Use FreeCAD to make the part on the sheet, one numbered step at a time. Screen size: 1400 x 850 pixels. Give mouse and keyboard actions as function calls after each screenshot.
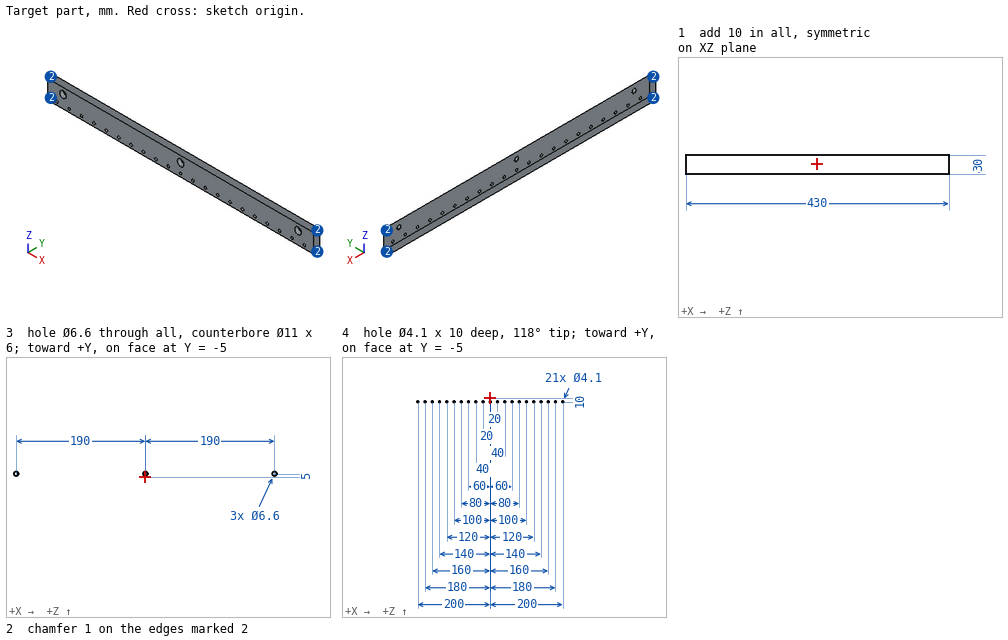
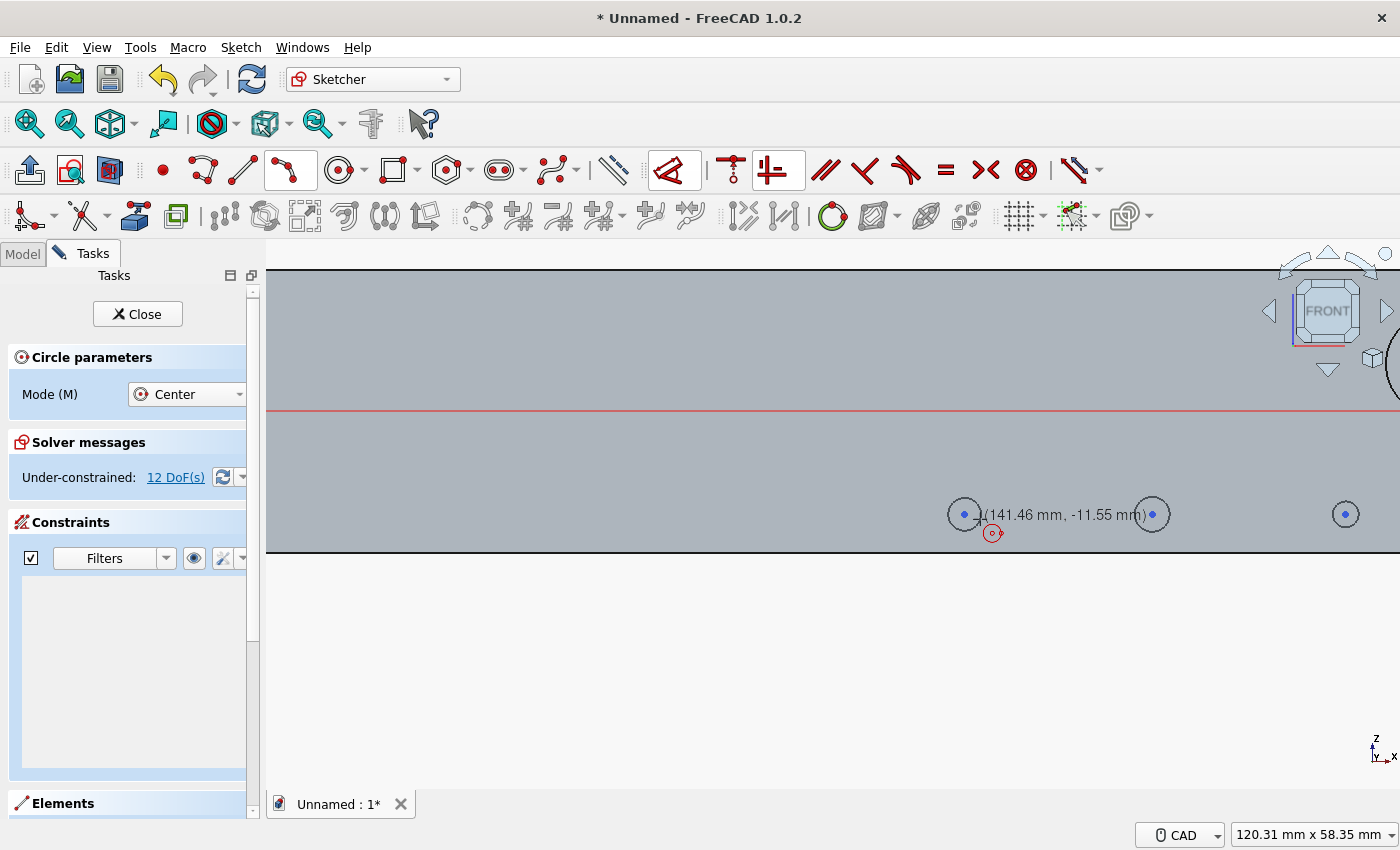
scroll(986, 523, down, 9)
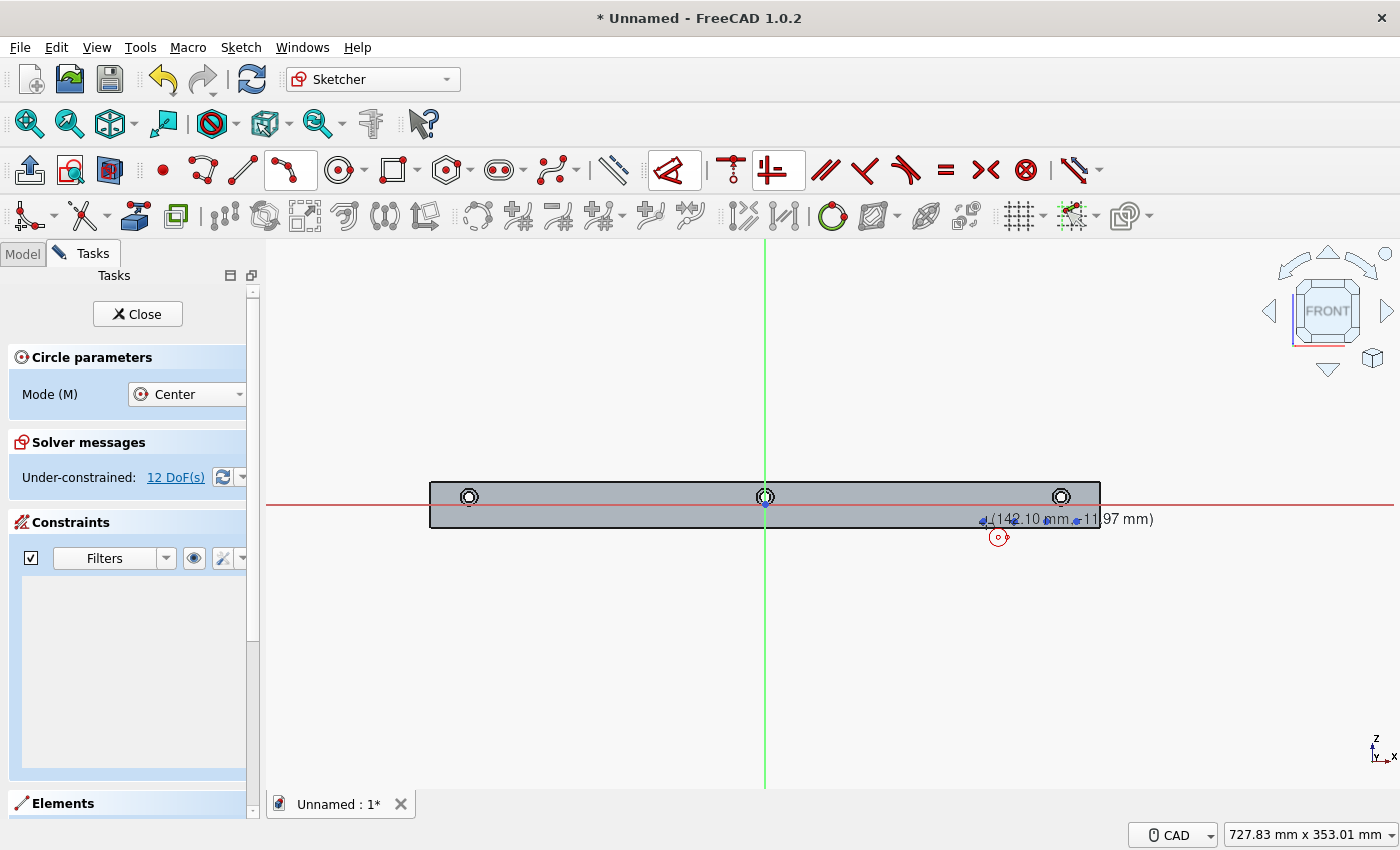
click(952, 521)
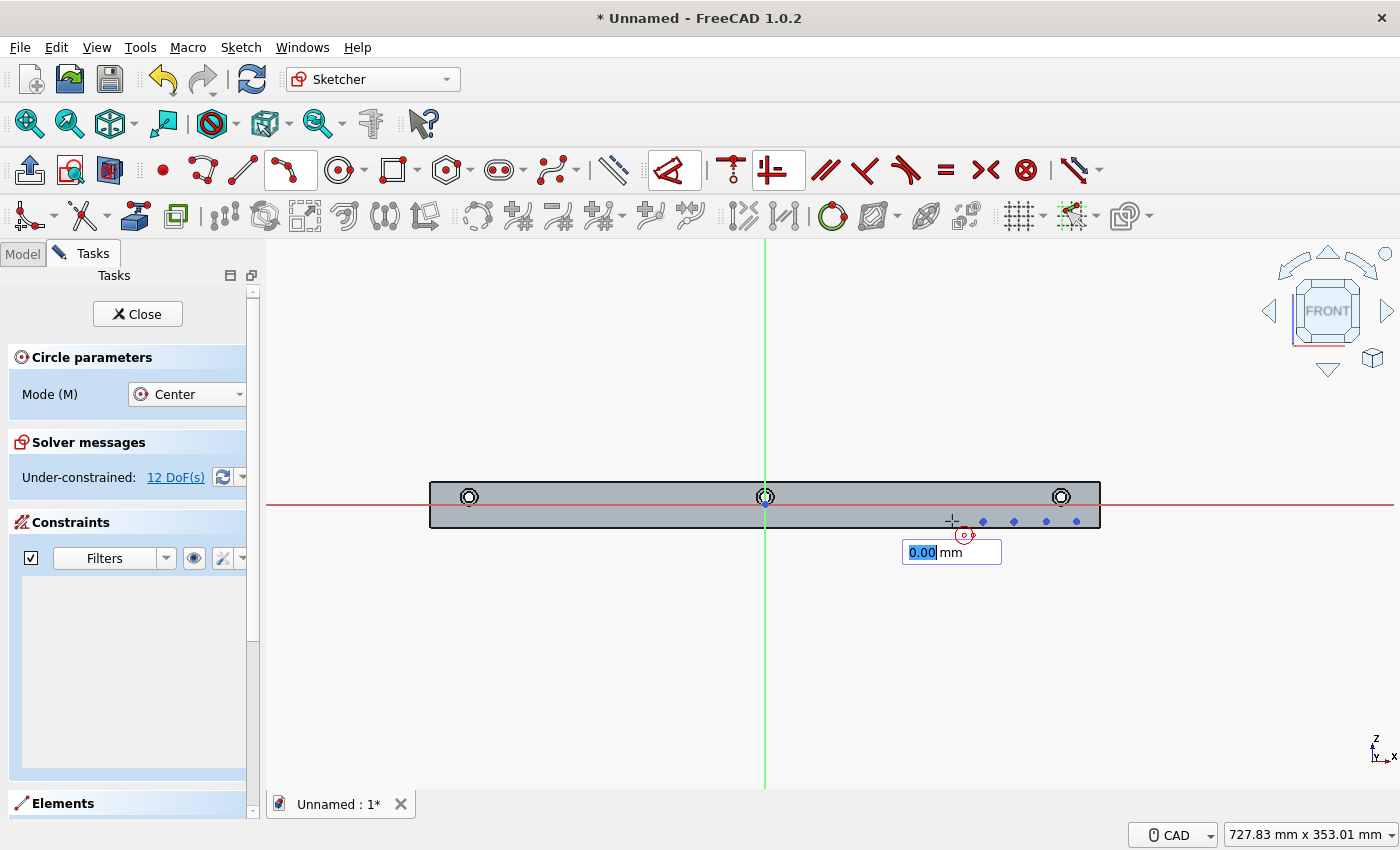
scroll(954, 523, up, 9)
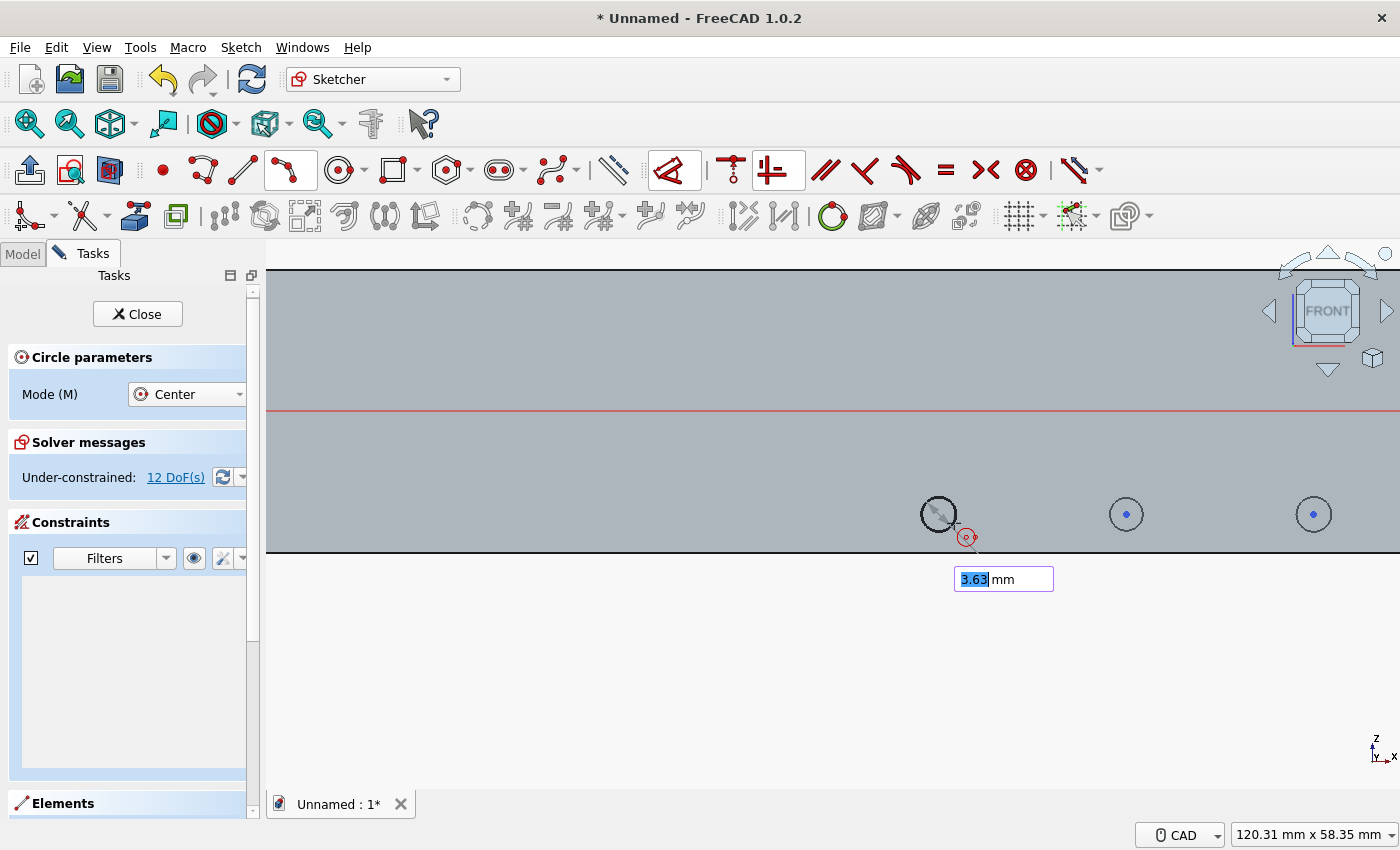
click(953, 519)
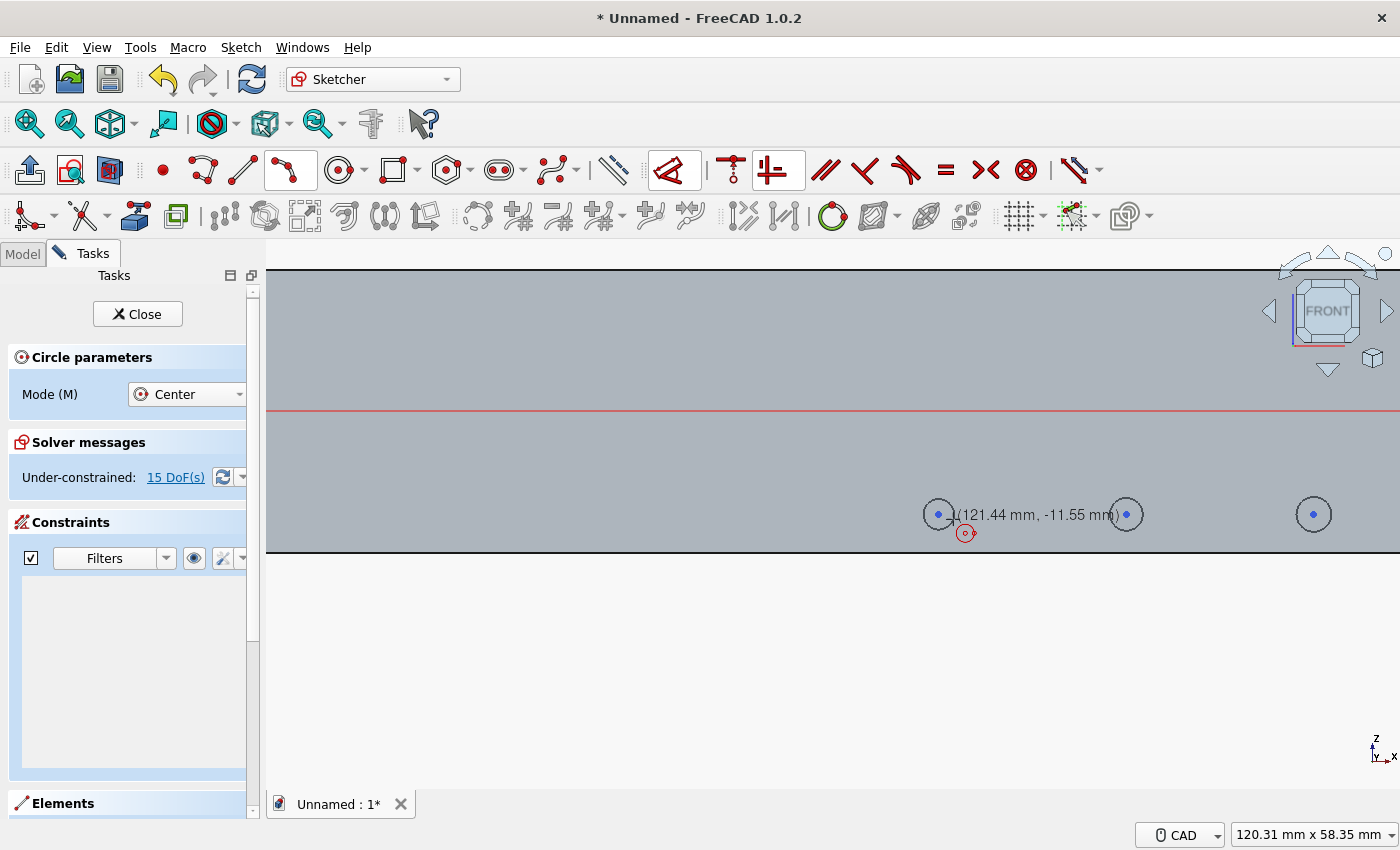
scroll(954, 523, down, 9)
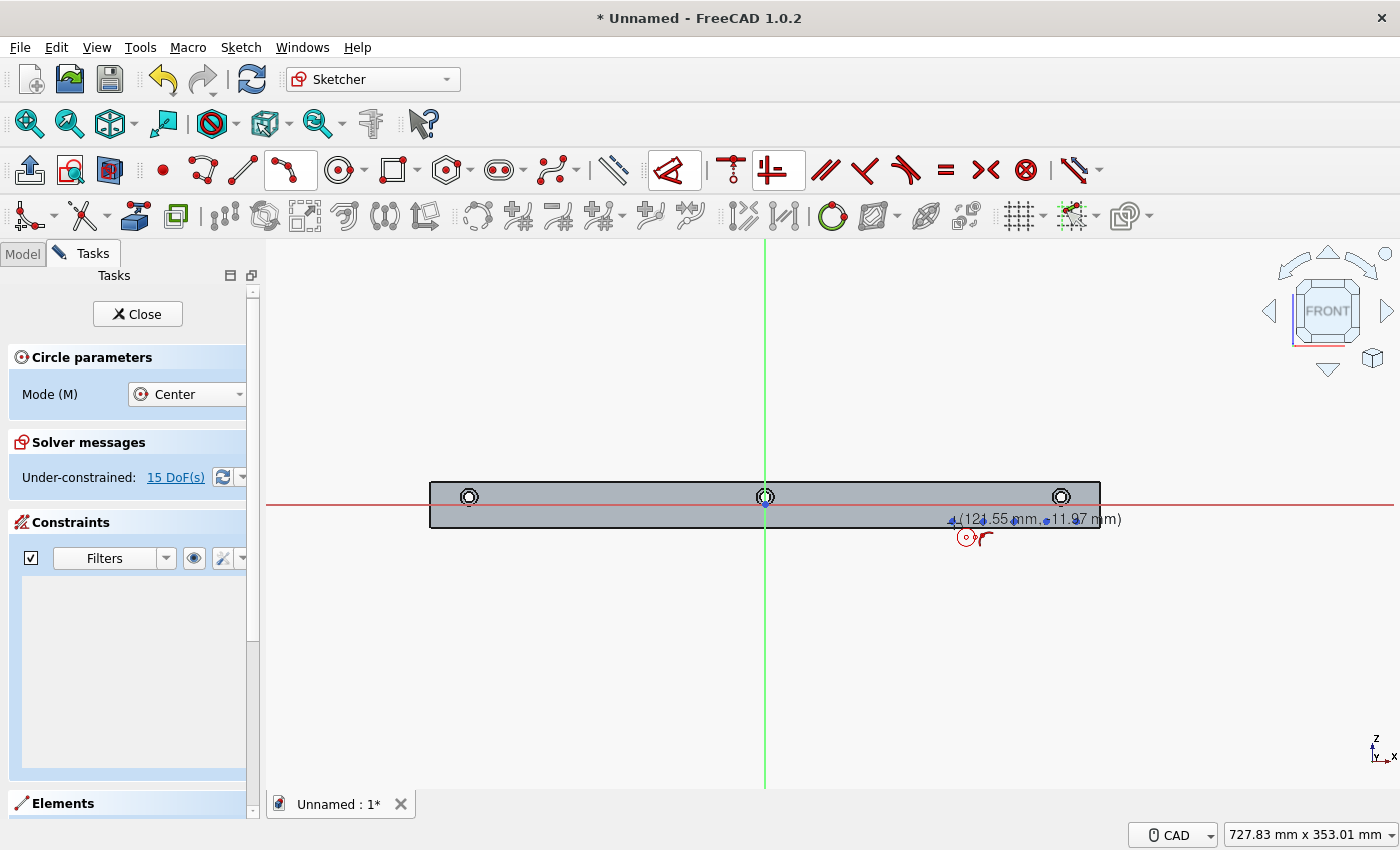
click(921, 521)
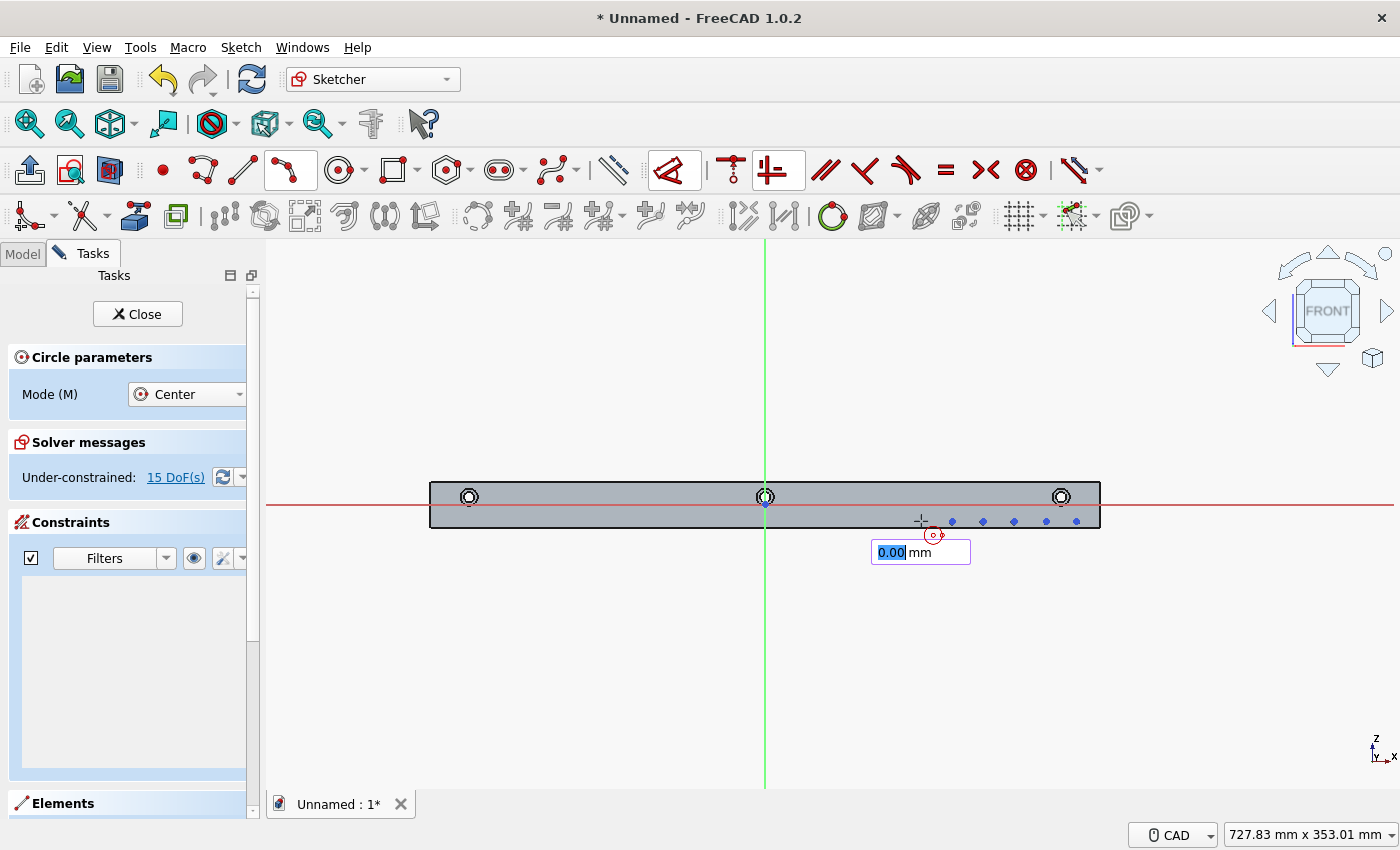
scroll(923, 523, up, 9)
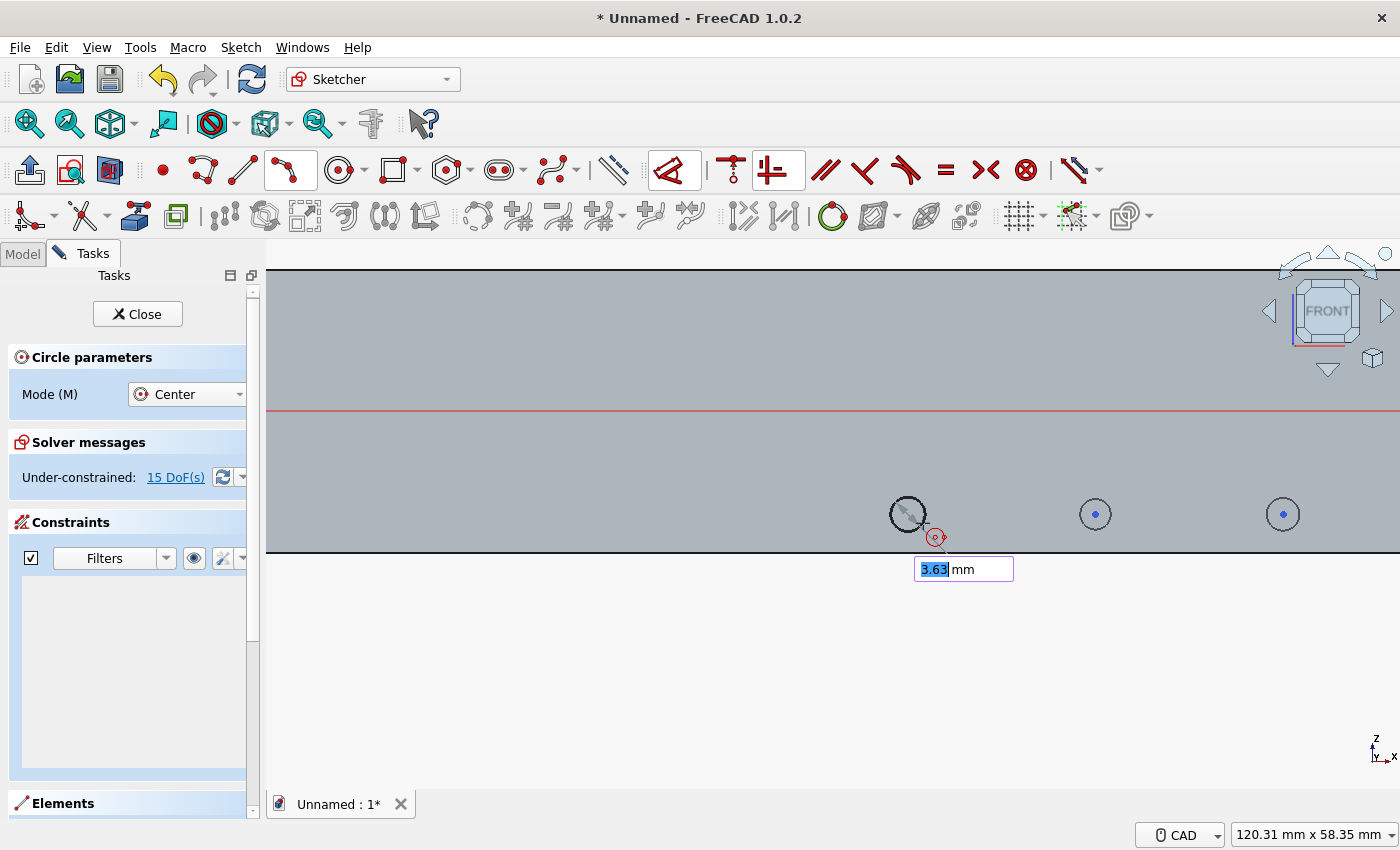
click(921, 519)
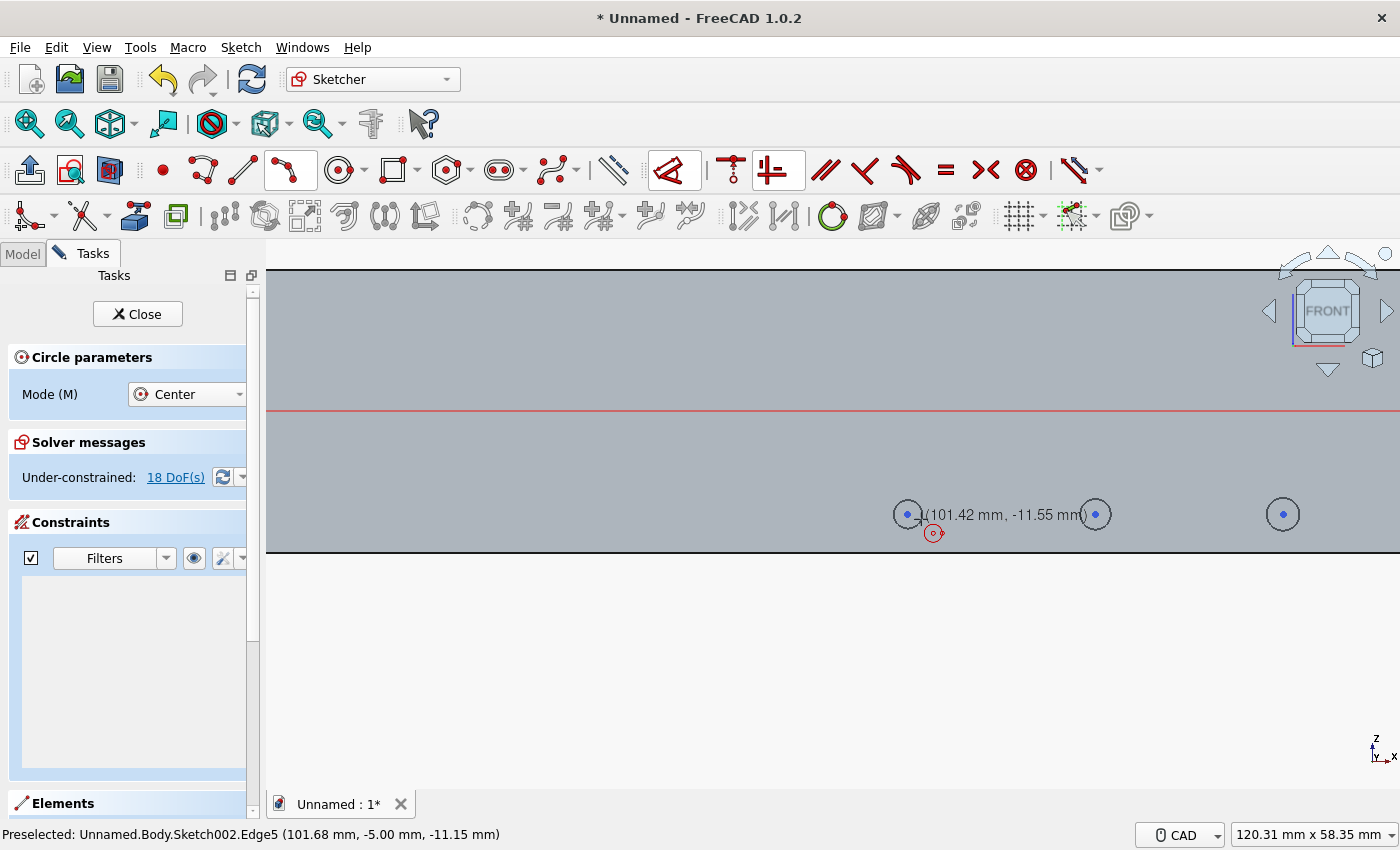
scroll(923, 523, down, 9)